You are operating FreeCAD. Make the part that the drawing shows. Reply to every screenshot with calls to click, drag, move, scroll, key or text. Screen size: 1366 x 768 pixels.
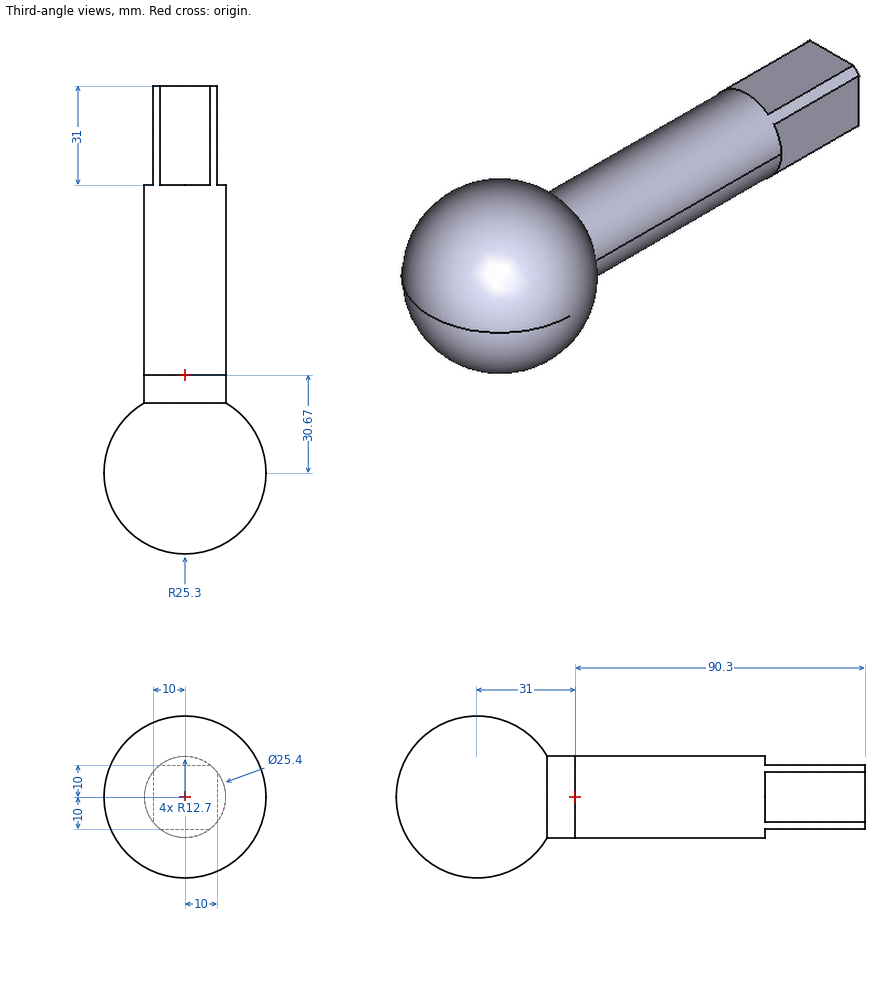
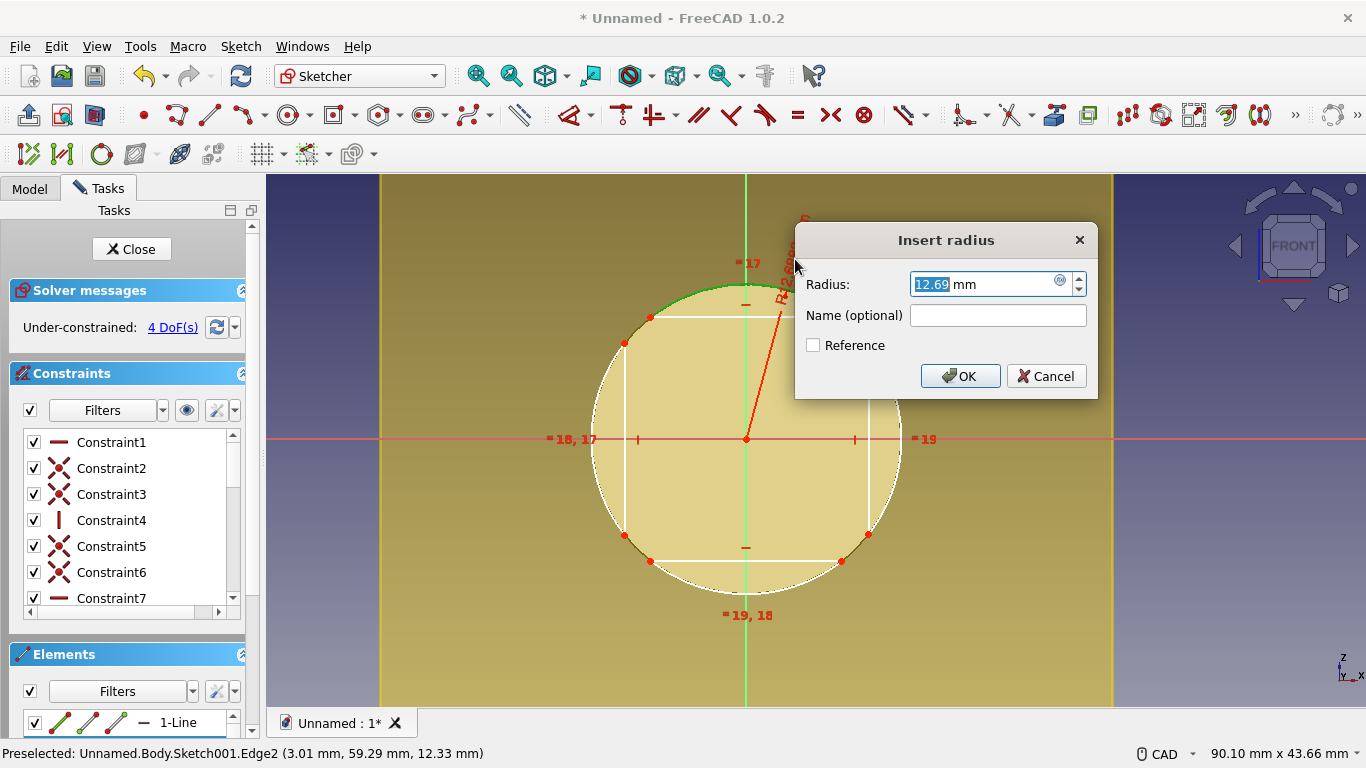
text(12.7)
key(Return)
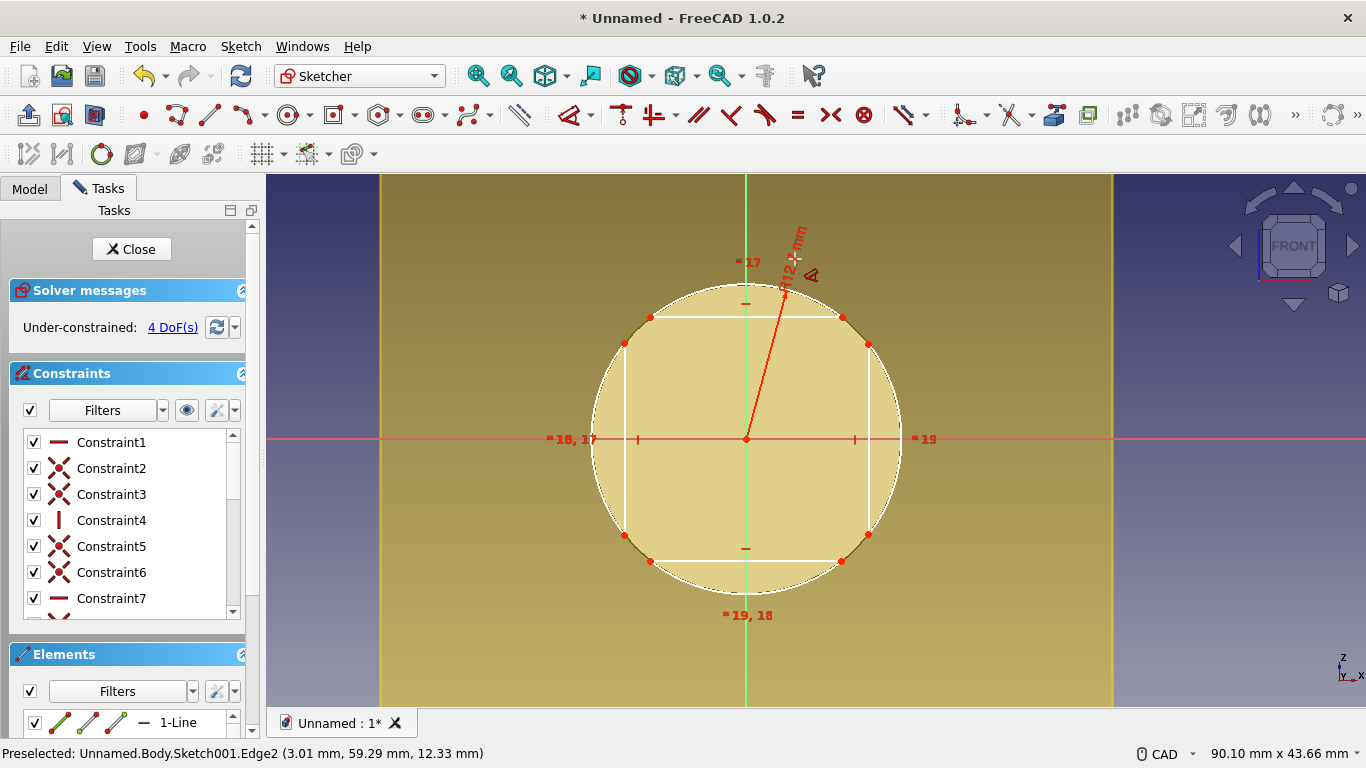
click(651, 317)
click(780, 378)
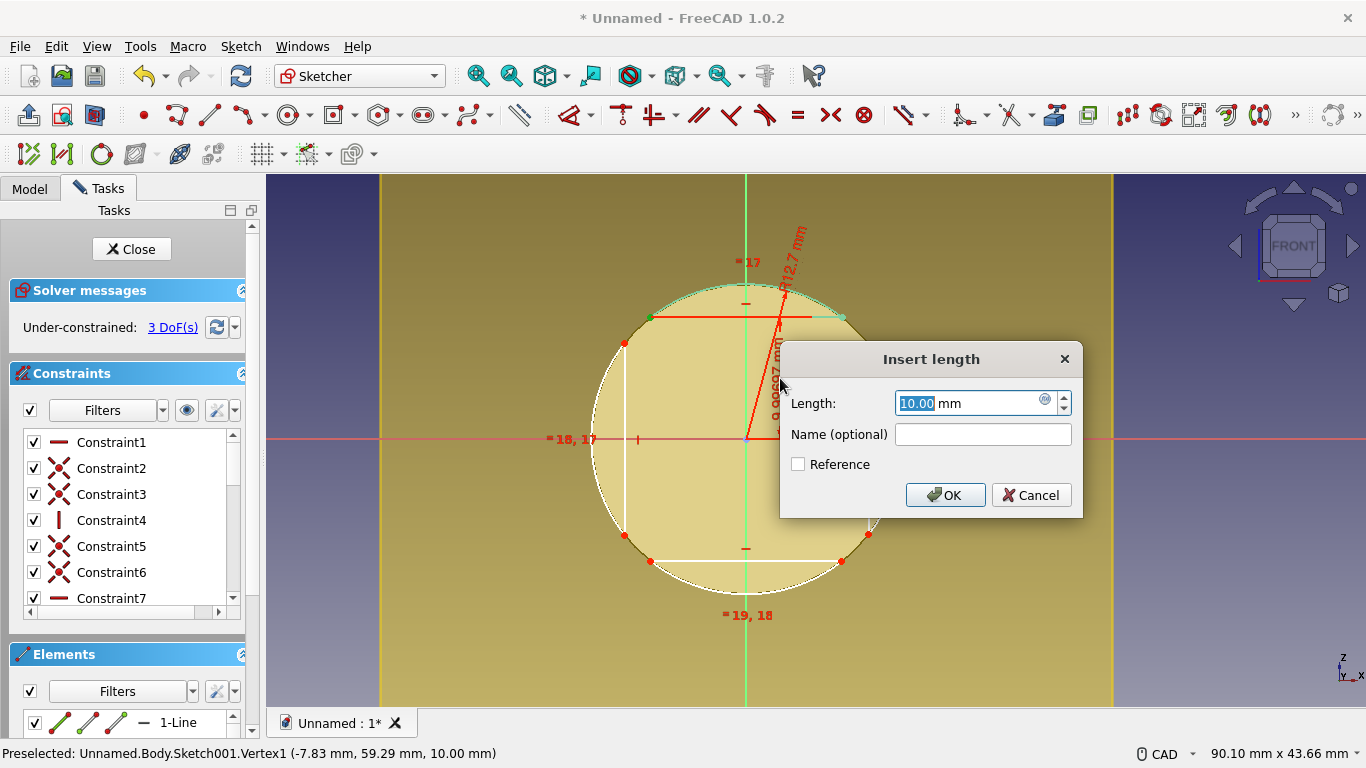
text(10)
key(Return)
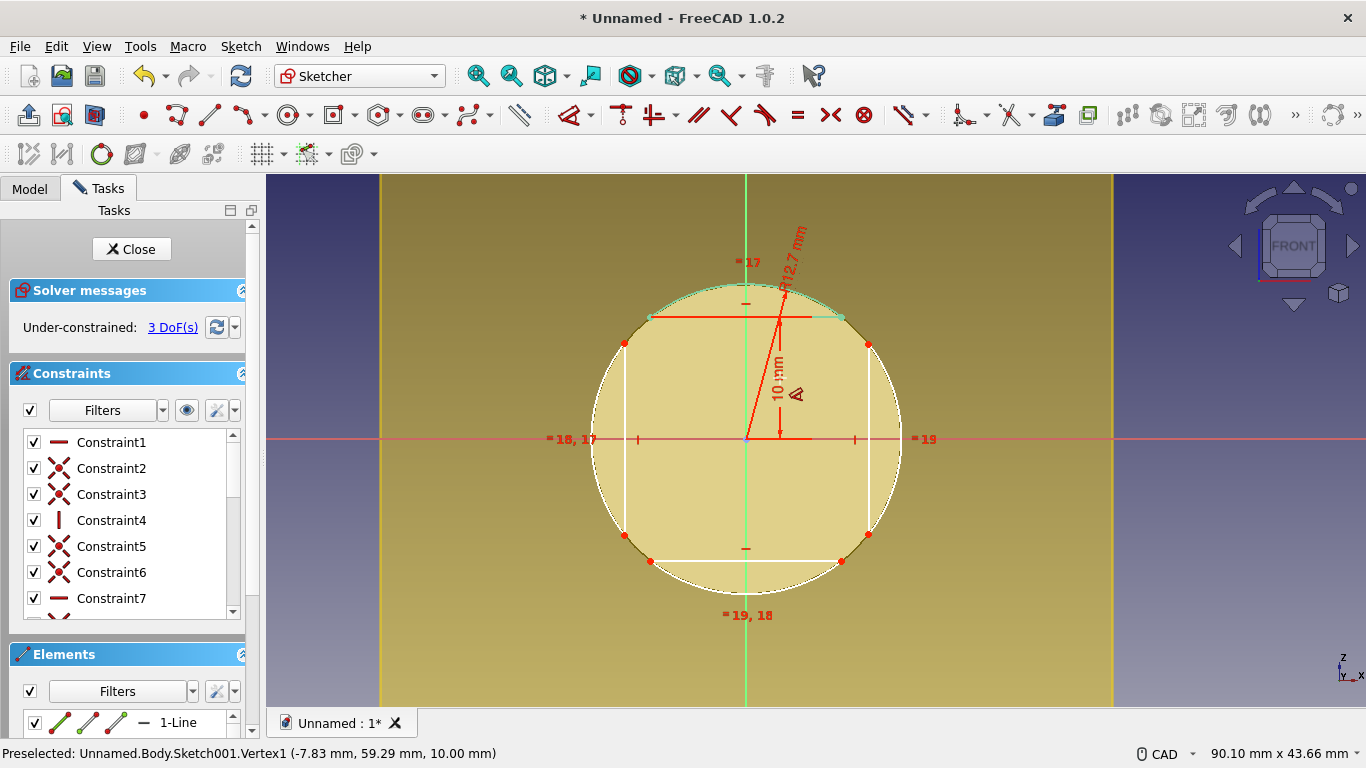
click(625, 343)
click(686, 473)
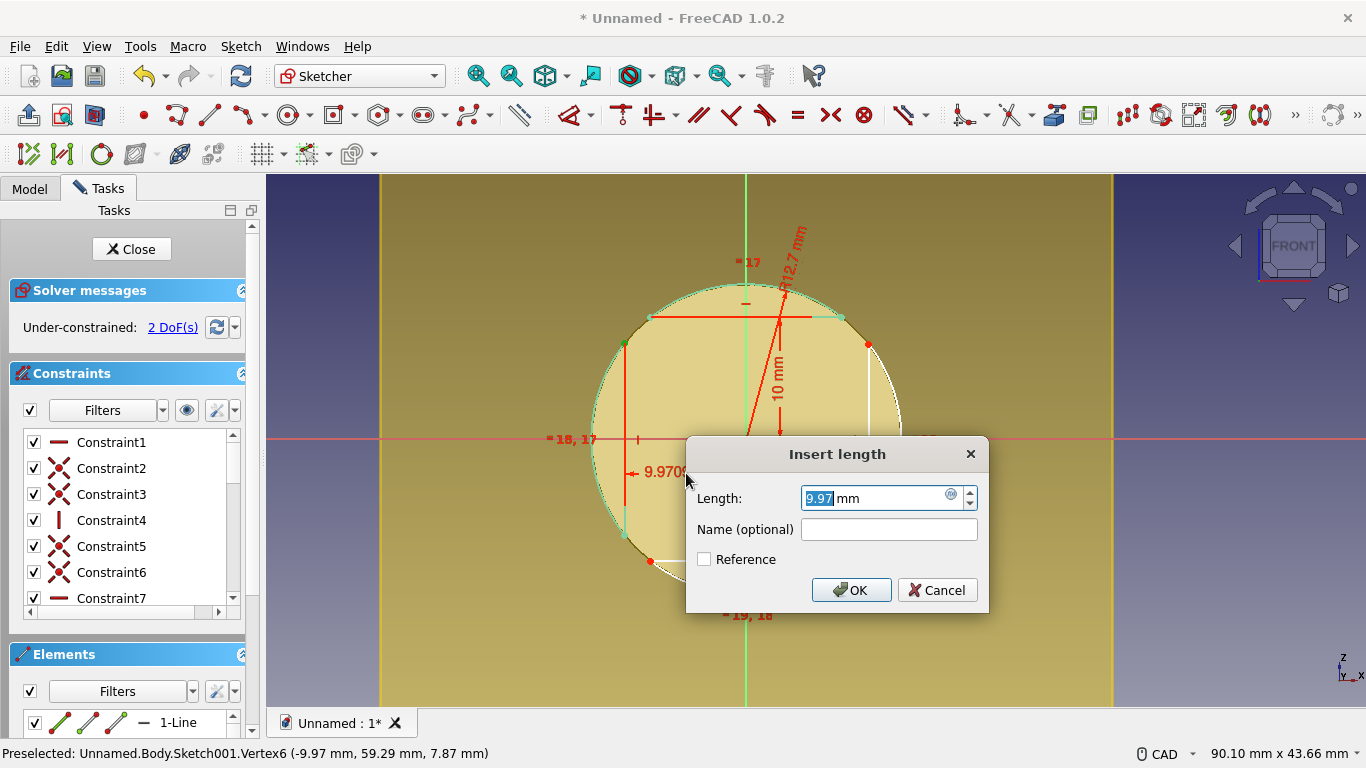
text(10)
key(Return)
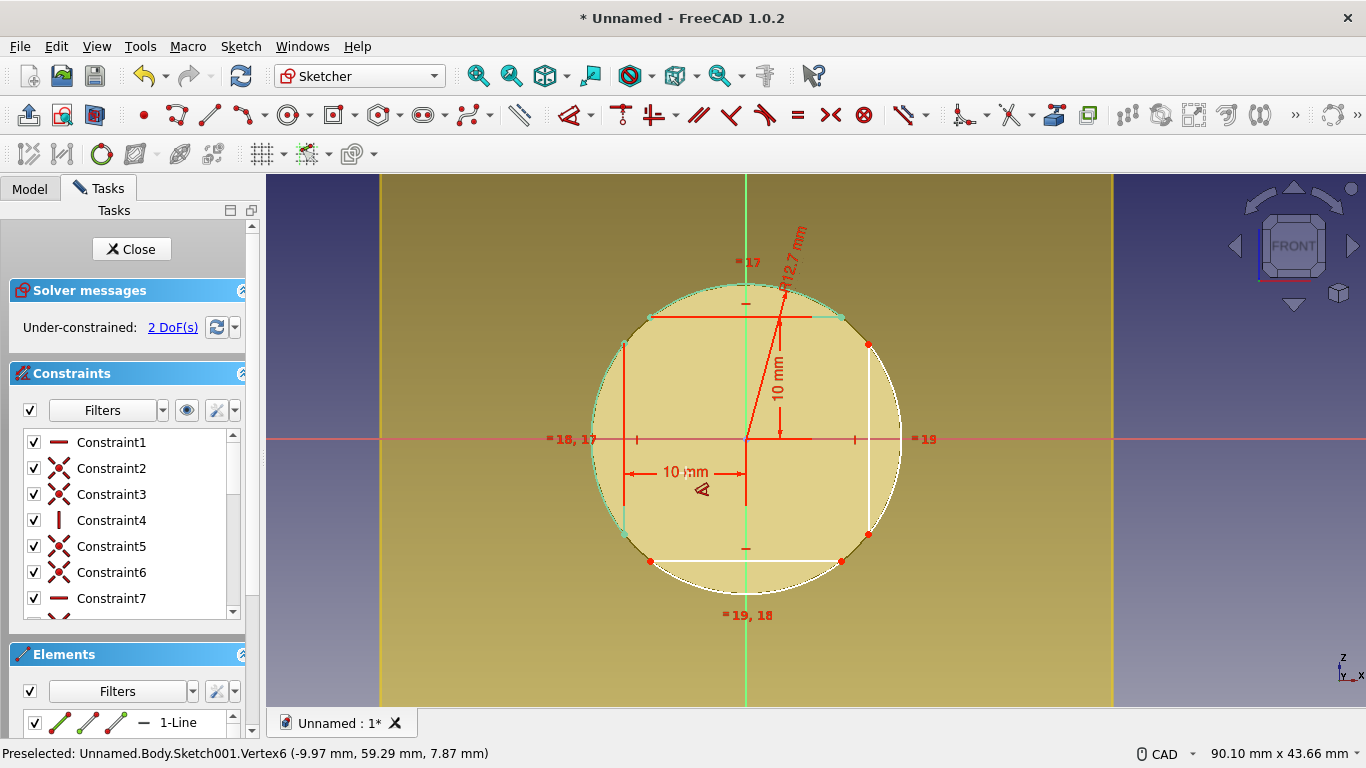
click(651, 561)
click(780, 500)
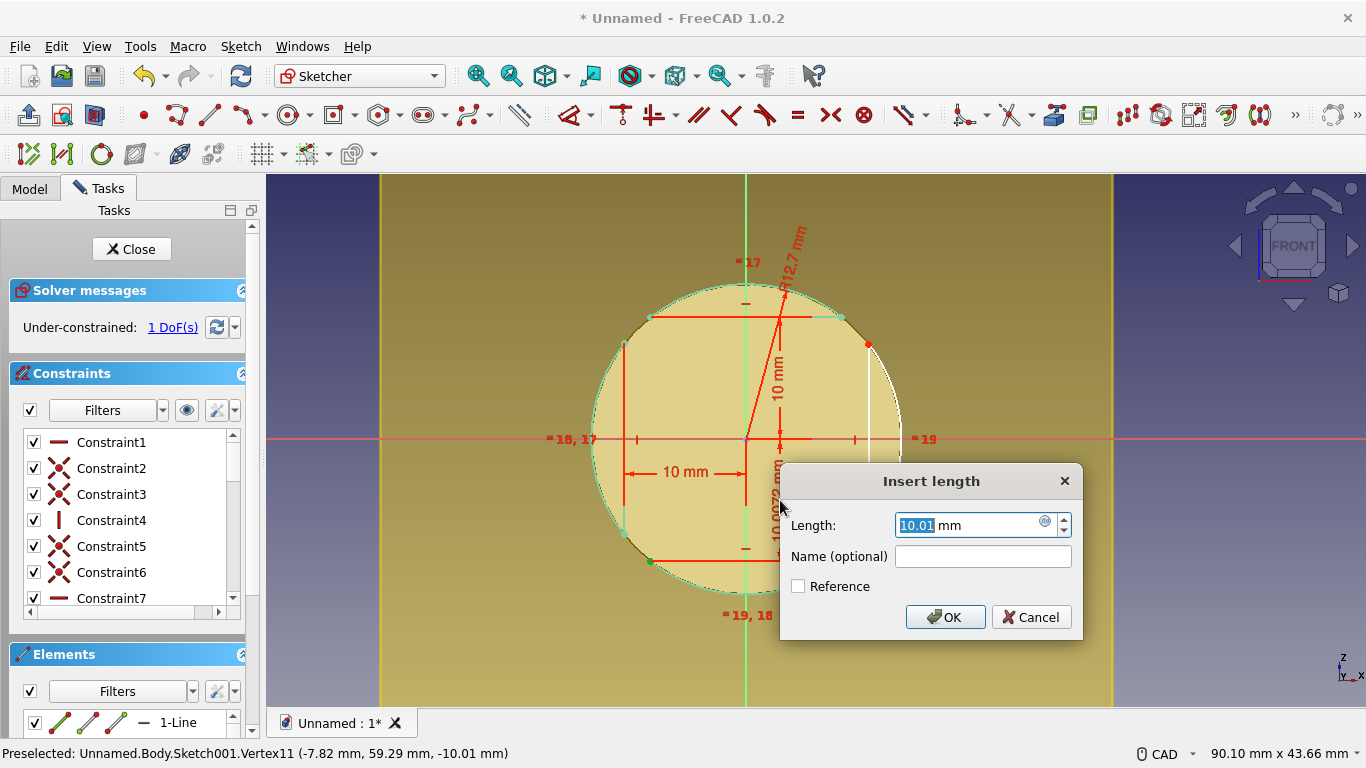
text(10)
key(Return)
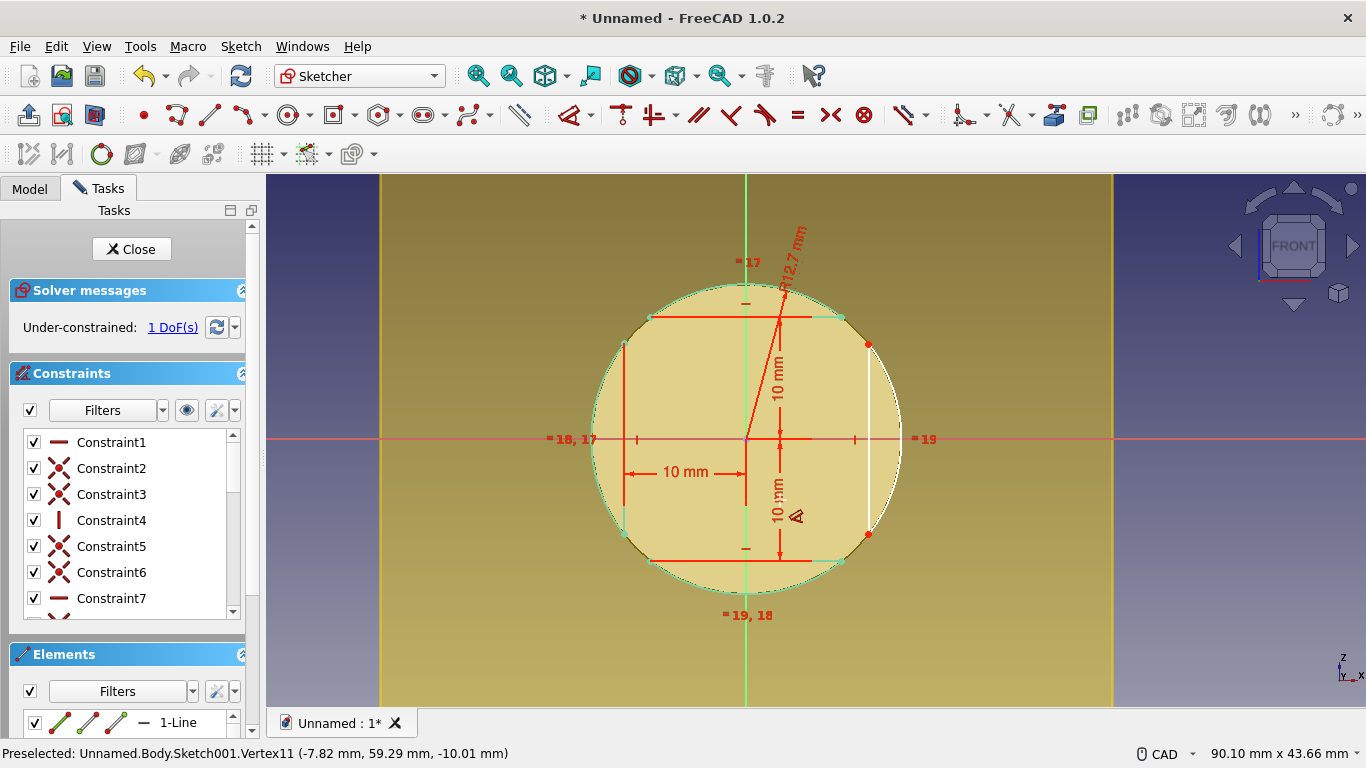
click(869, 534)
click(808, 405)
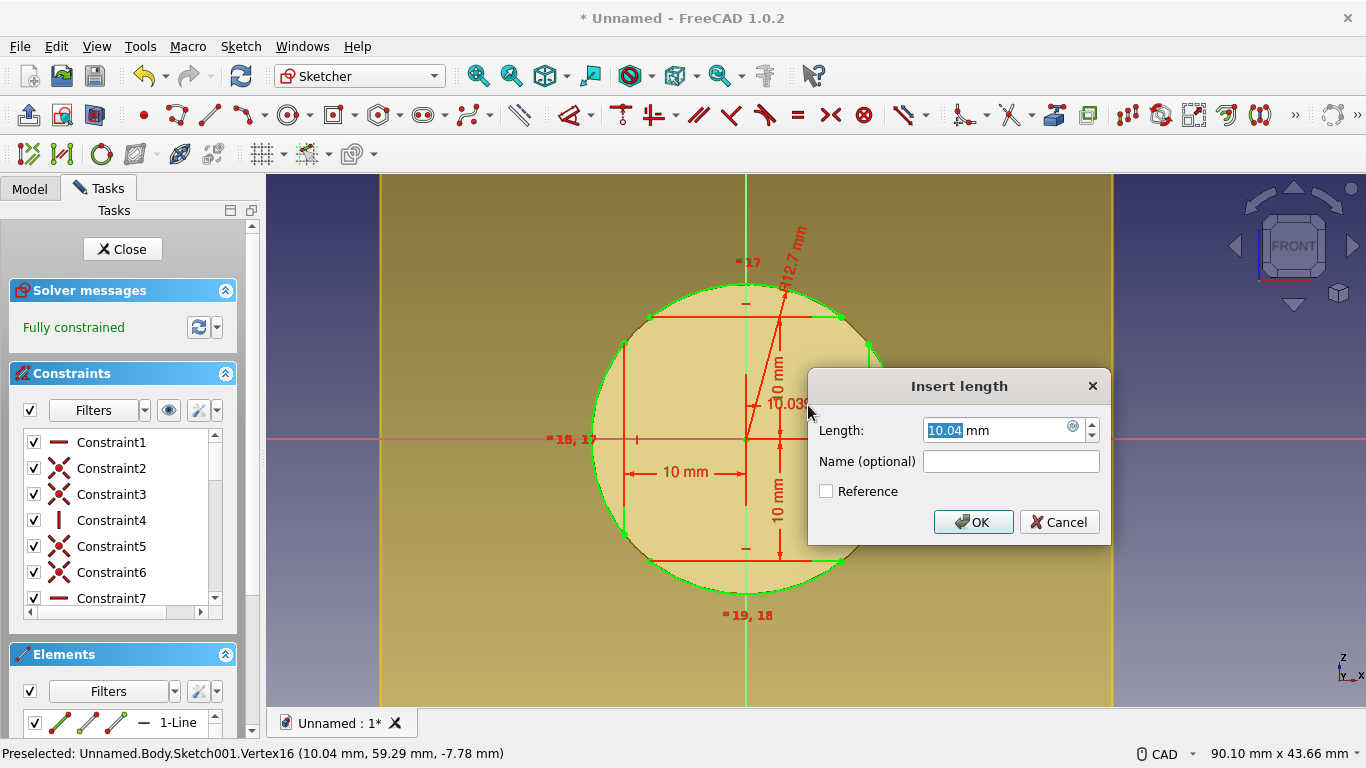
text(10)
key(Return)
key(Escape)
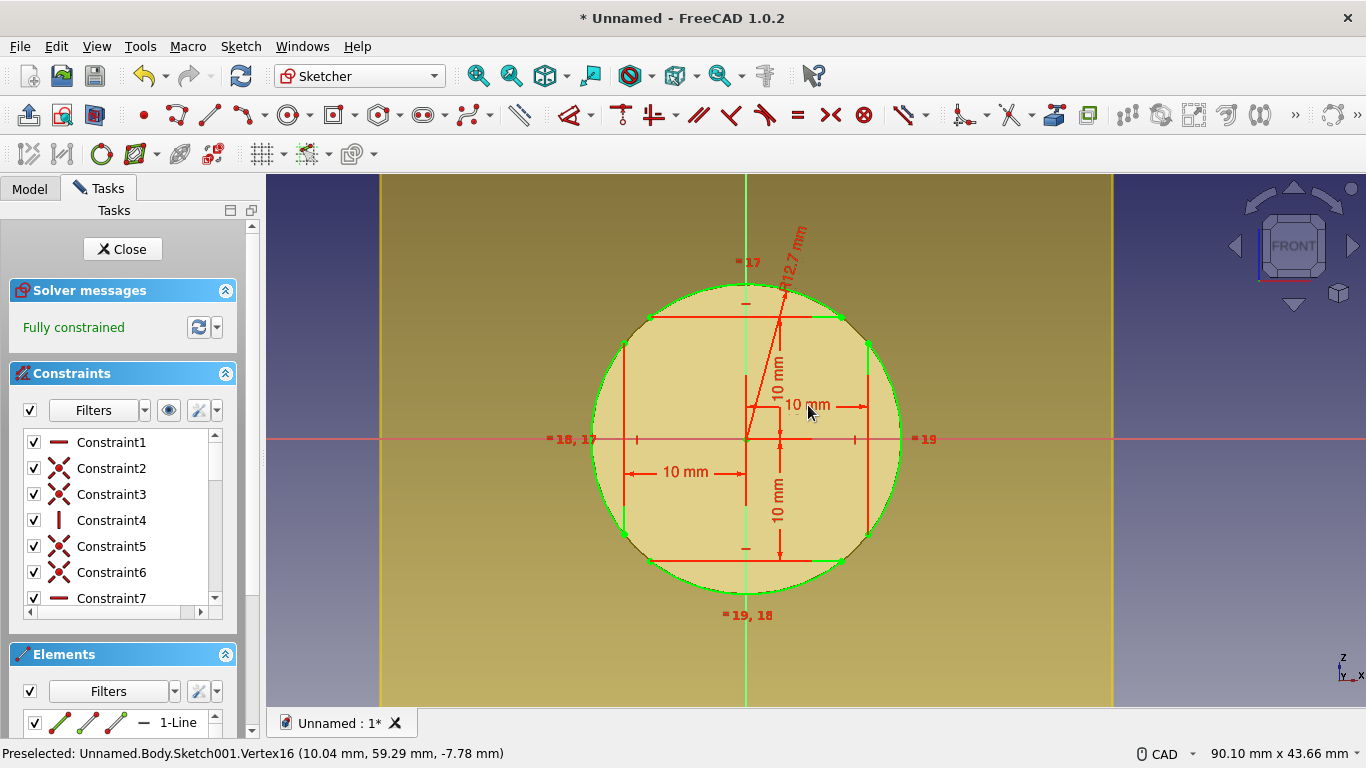
click(123, 249)